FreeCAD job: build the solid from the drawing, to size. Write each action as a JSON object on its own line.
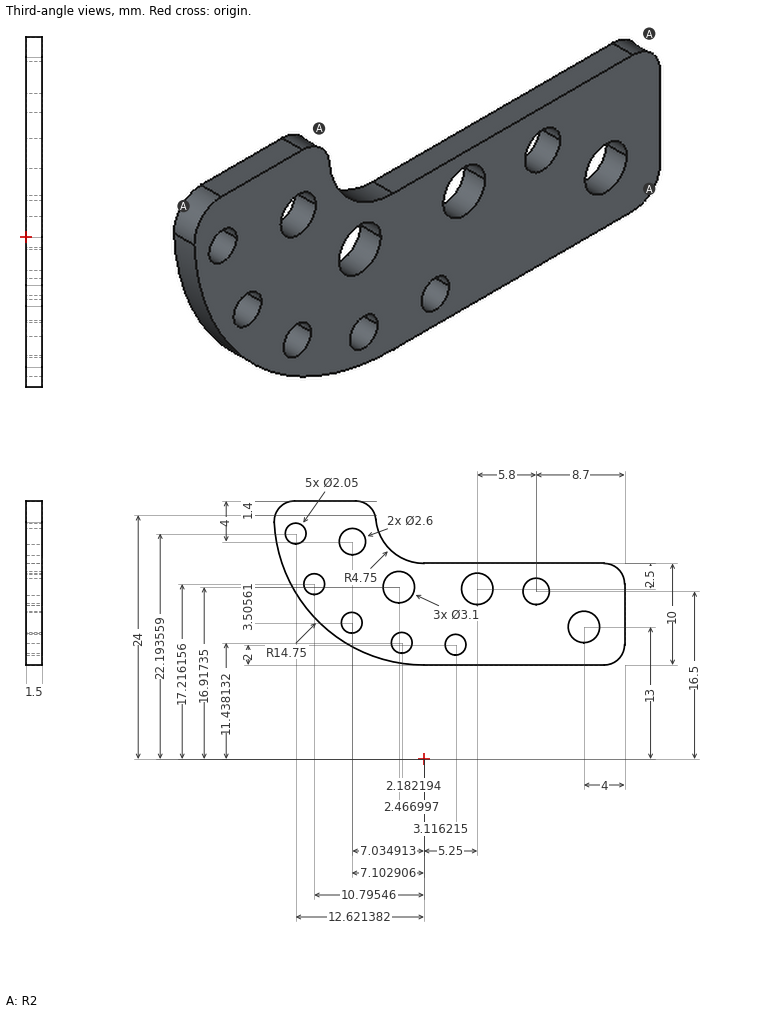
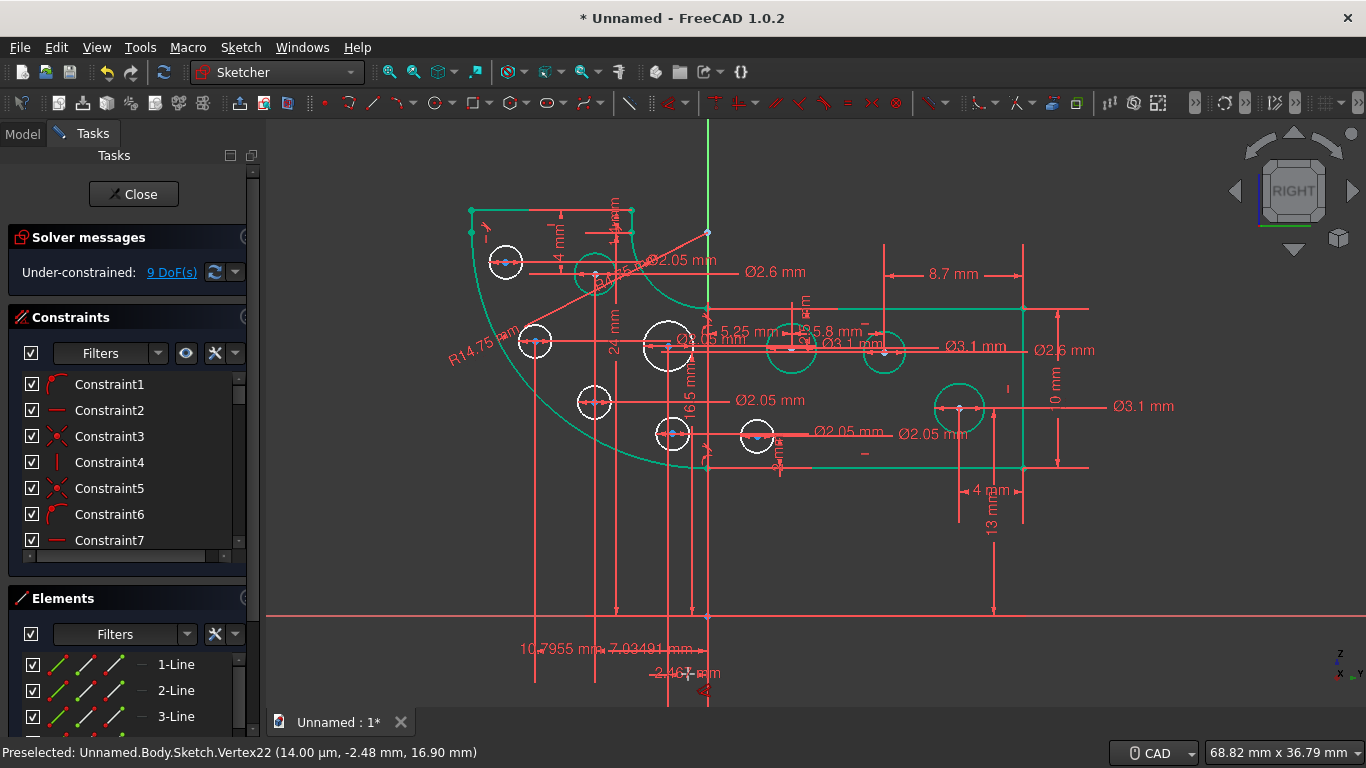
{"action": "left_click", "coordinate": [668, 346]}
{"action": "left_click", "coordinate": [634, 481]}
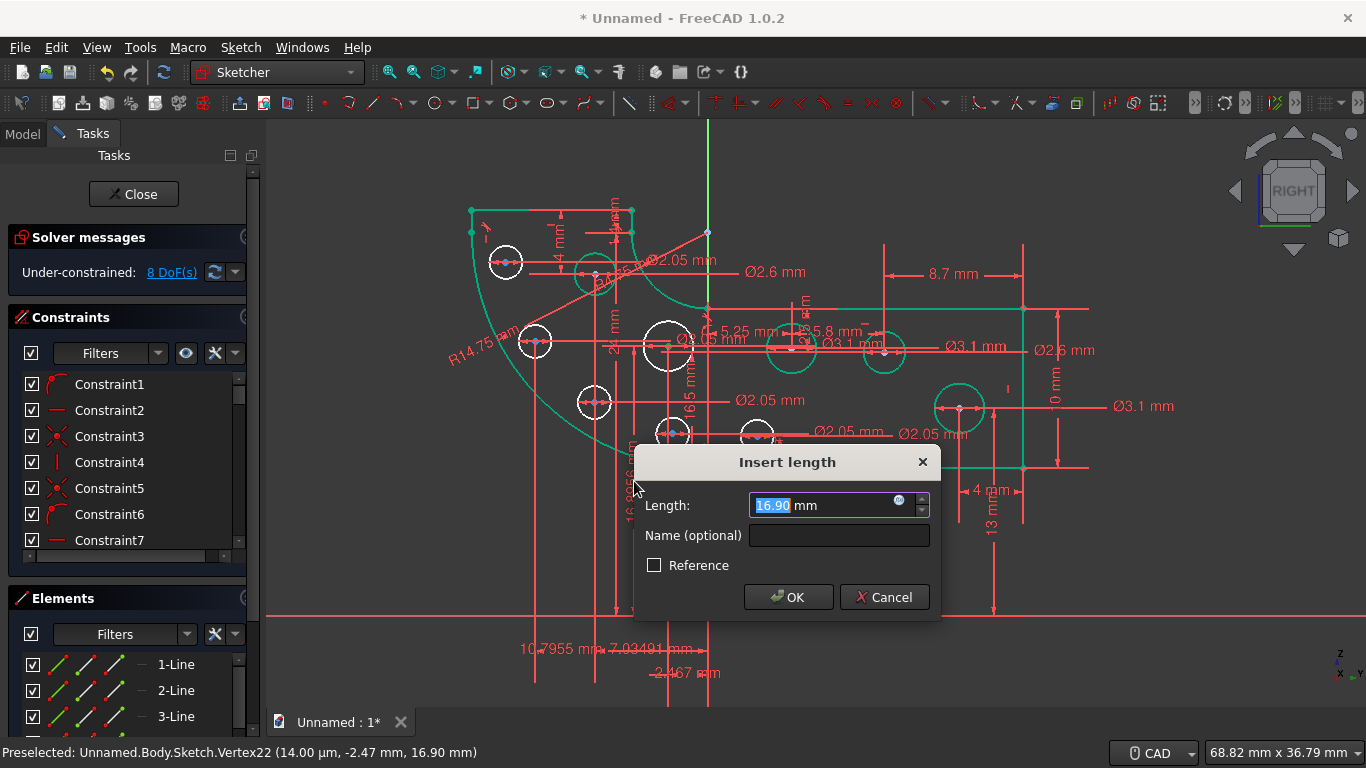
{"action": "type", "text": "16.91735"}
{"action": "key", "text": "Return"}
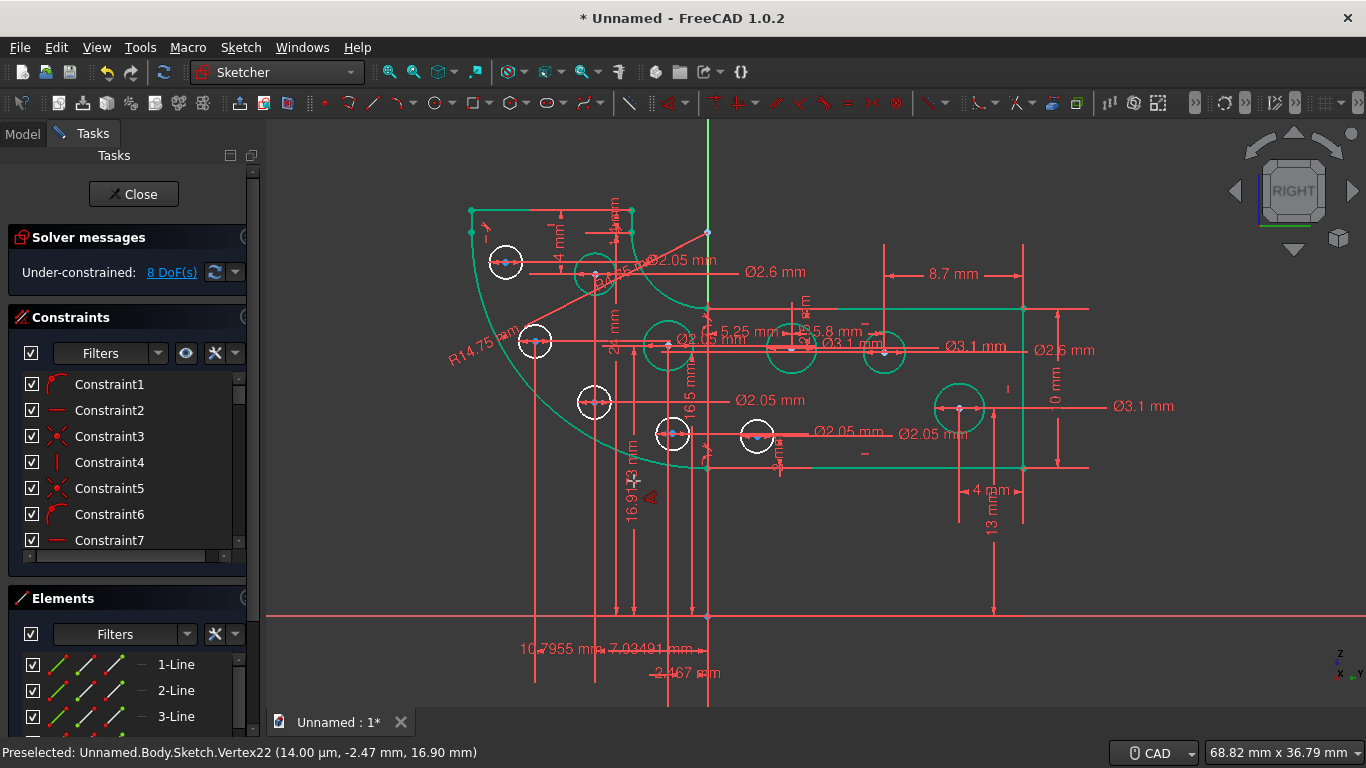
{"action": "left_click", "coordinate": [594, 402]}
{"action": "left_click", "coordinate": [625, 368]}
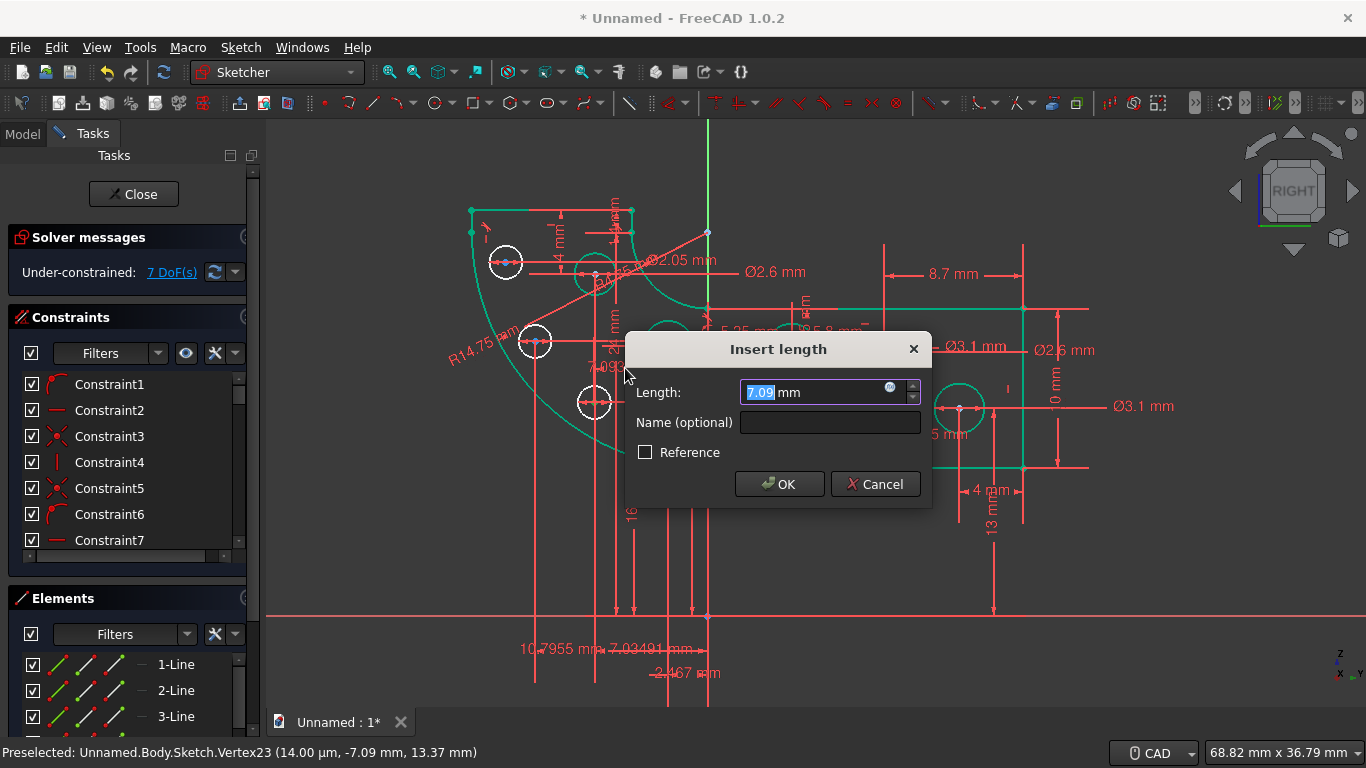
{"action": "type", "text": "7.102906"}
{"action": "key", "text": "Return"}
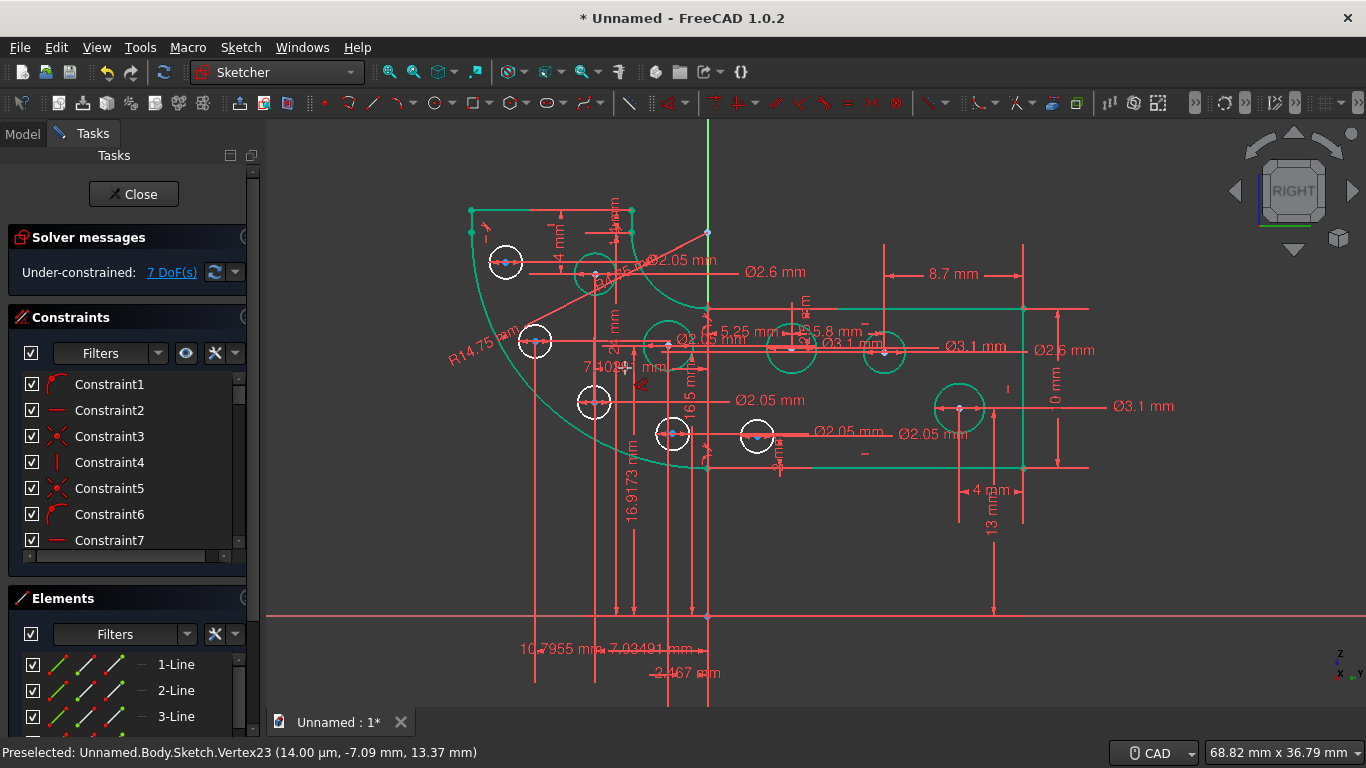
{"action": "left_click", "coordinate": [673, 434]}
{"action": "left_click", "coordinate": [690, 254]}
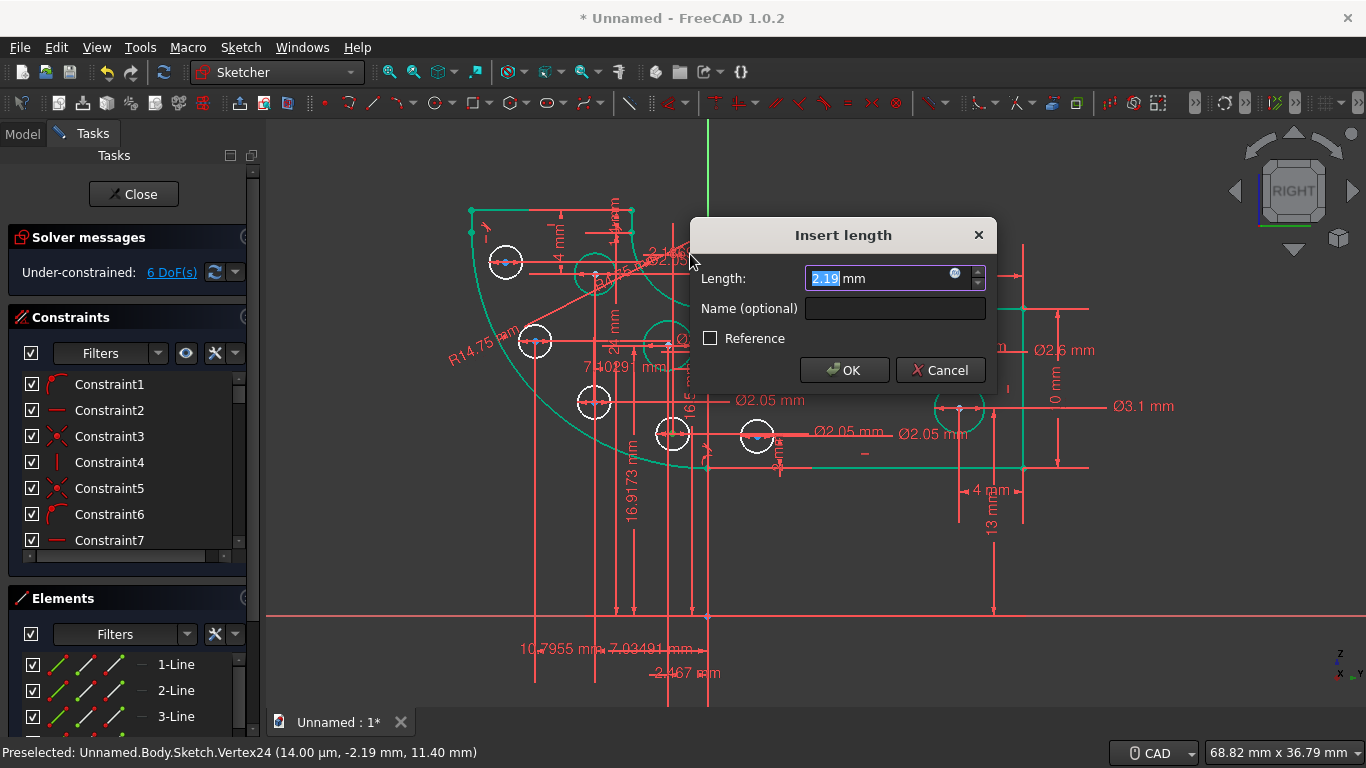
{"action": "type", "text": "2.182194"}
{"action": "key", "text": "Return"}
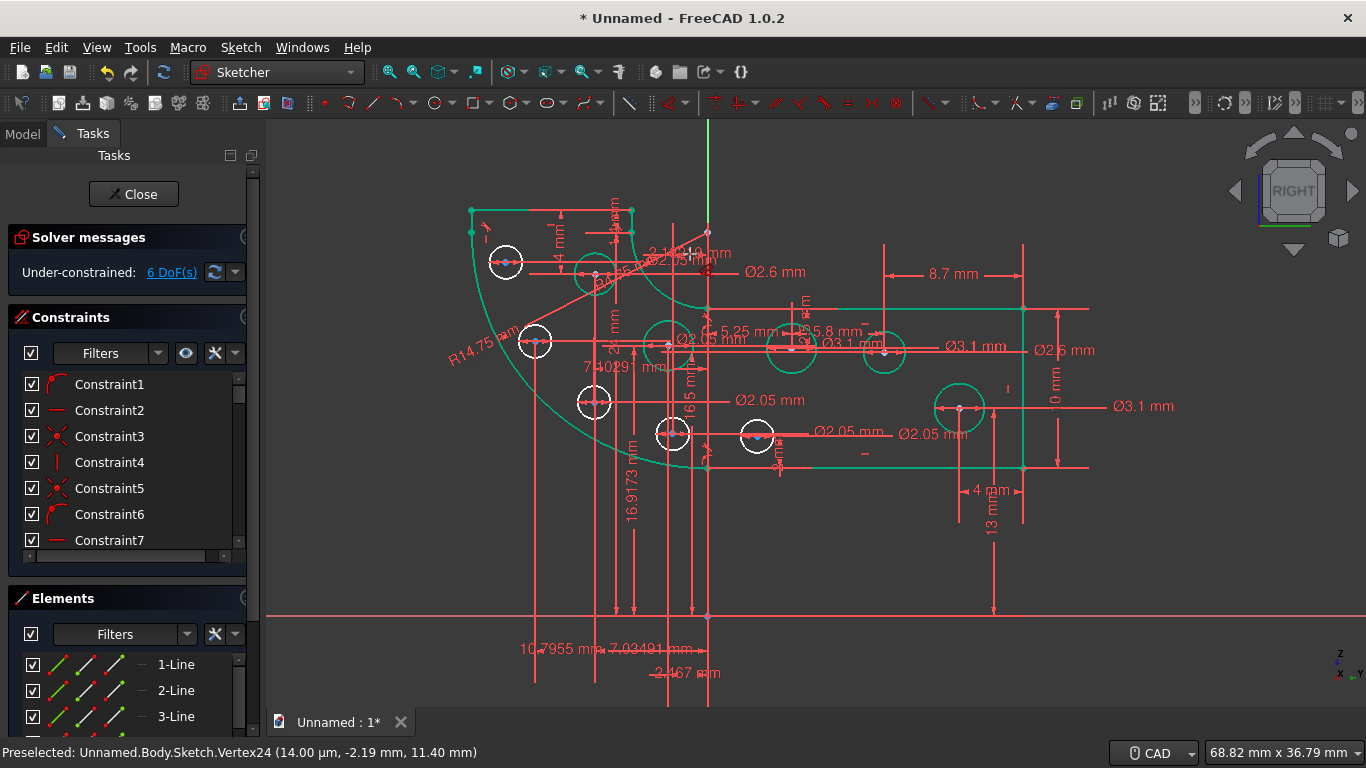
{"action": "left_click", "coordinate": [757, 436]}
{"action": "left_click", "coordinate": [732, 650]}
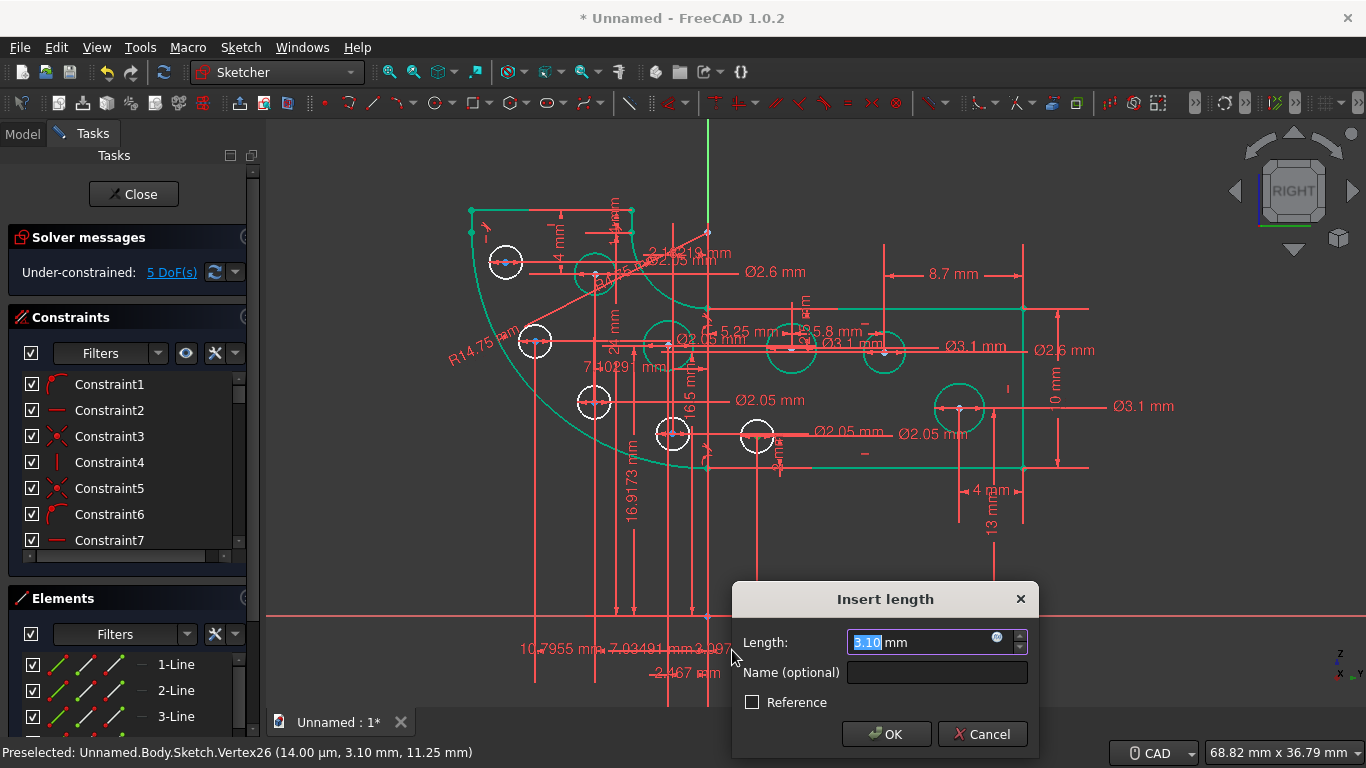
{"action": "type", "text": "3.116215"}
{"action": "key", "text": "Return"}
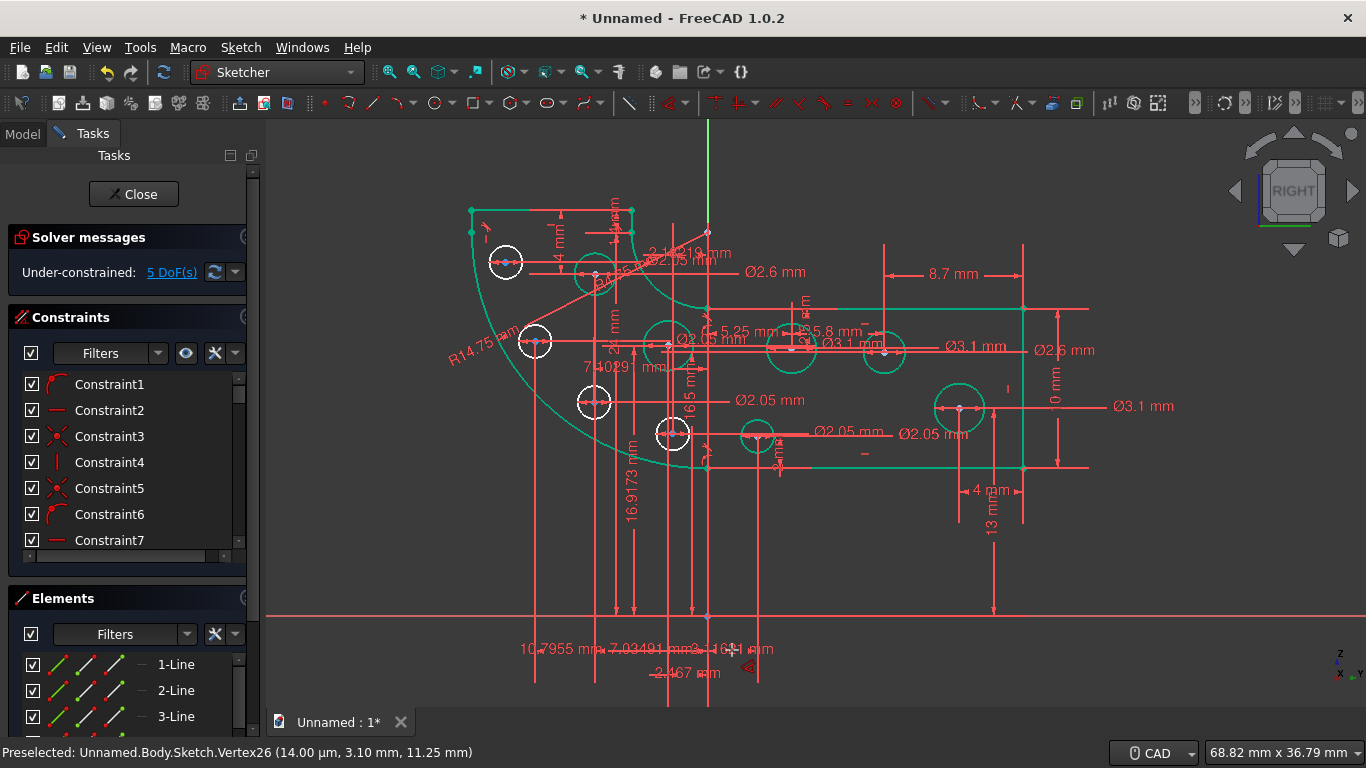
{"action": "left_click", "coordinate": [668, 346]}